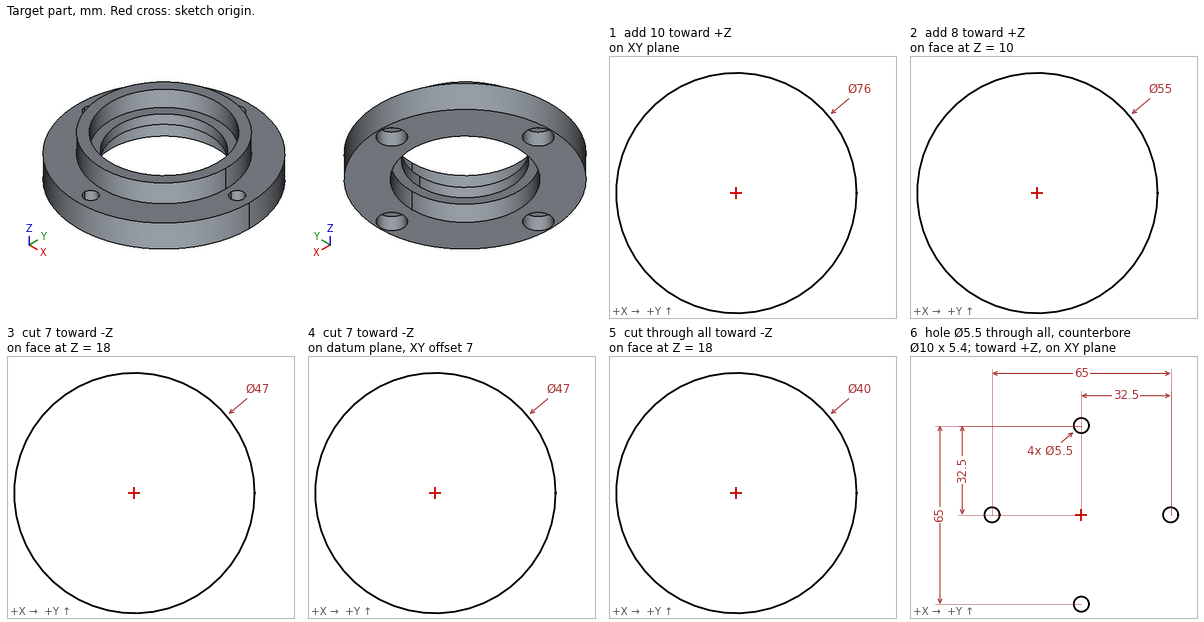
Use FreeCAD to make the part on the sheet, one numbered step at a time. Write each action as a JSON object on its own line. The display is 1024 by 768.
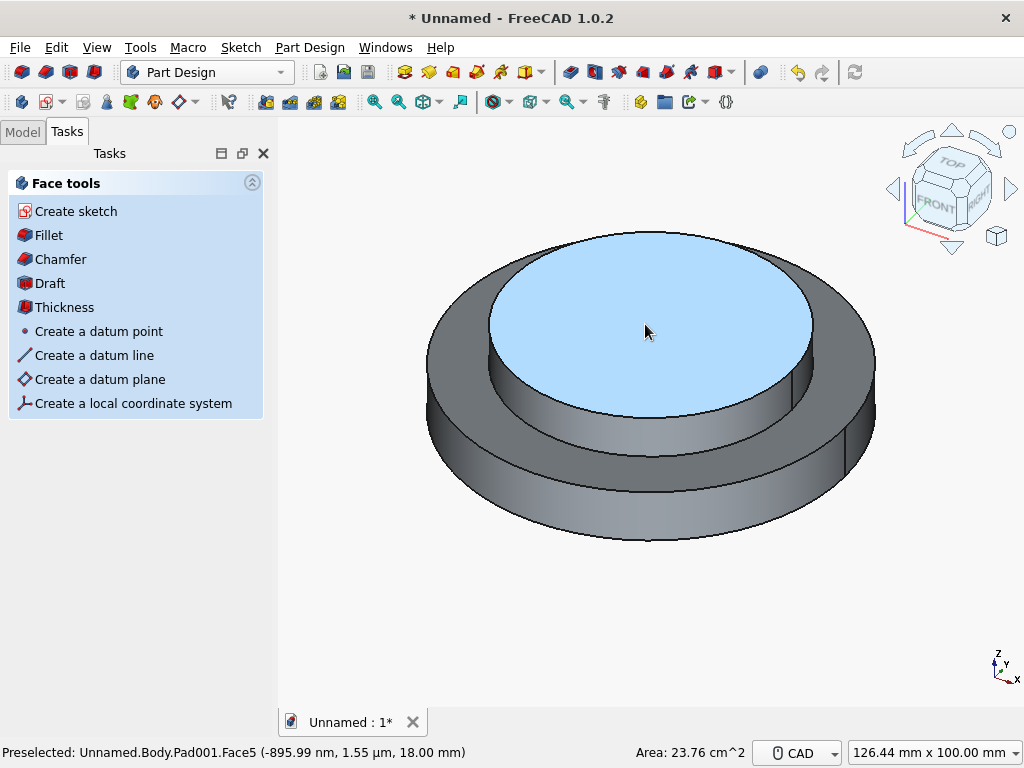
{"action": "left_click", "coordinate": [46, 102]}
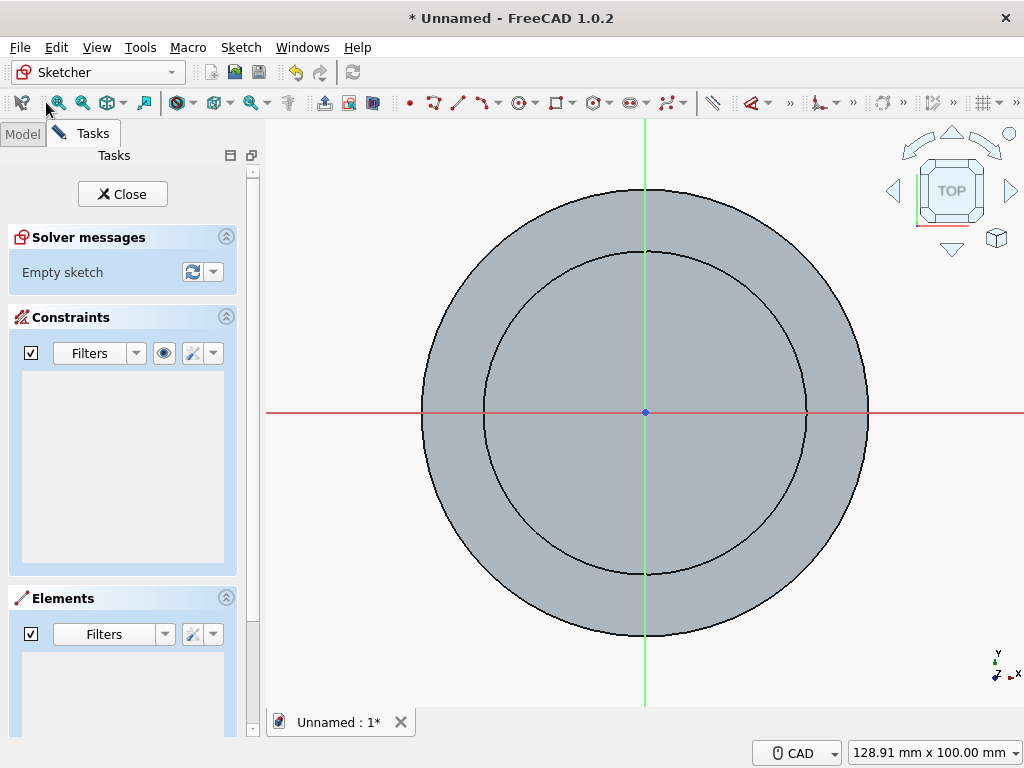
{"action": "scroll", "coordinate": [784, 413], "scroll_direction": "up", "scroll_amount": 2}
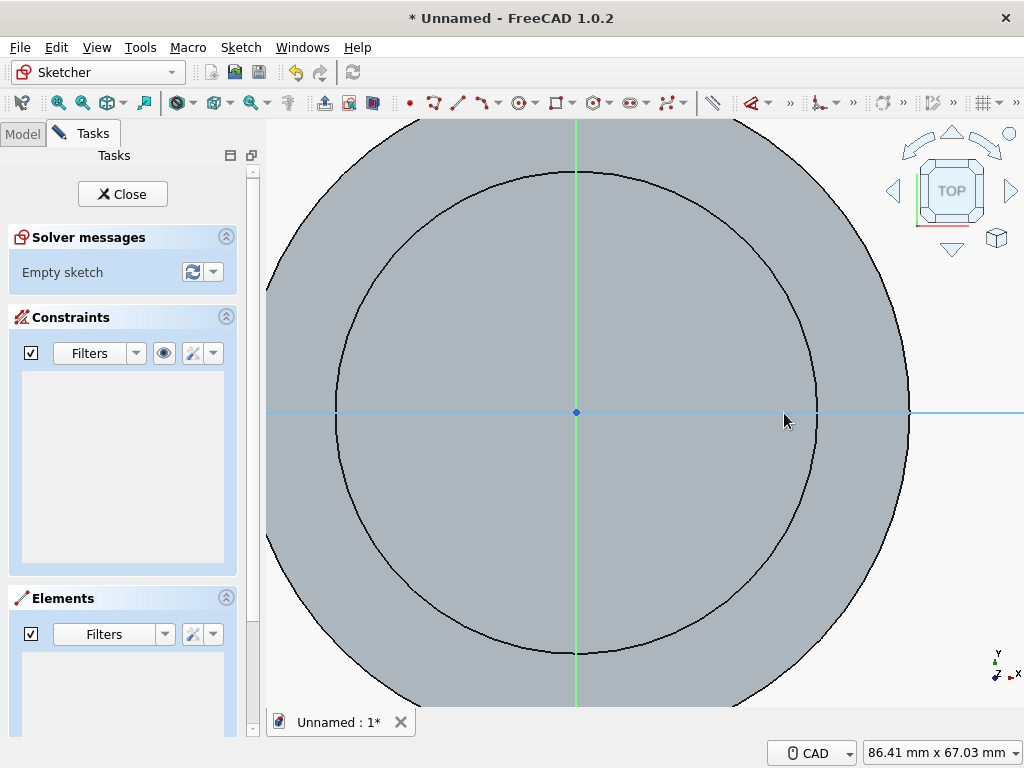
{"action": "key", "text": "g c"}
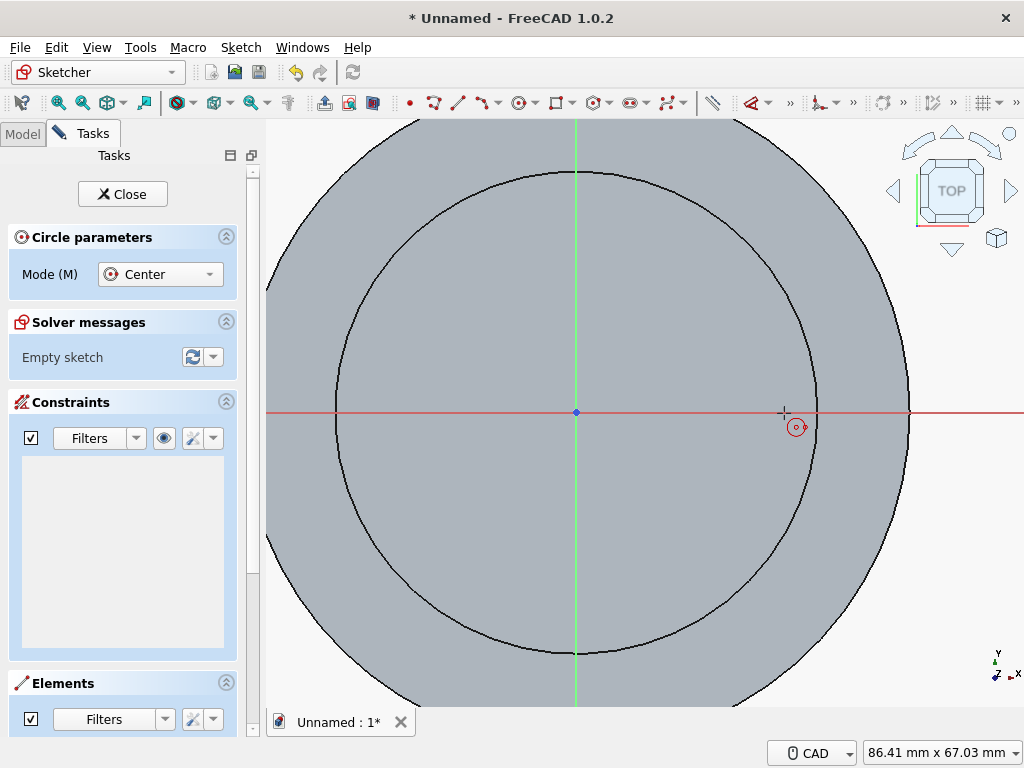
{"action": "left_click", "coordinate": [576, 413]}
{"action": "left_click", "coordinate": [722, 267]}
{"action": "key", "text": "Escape"}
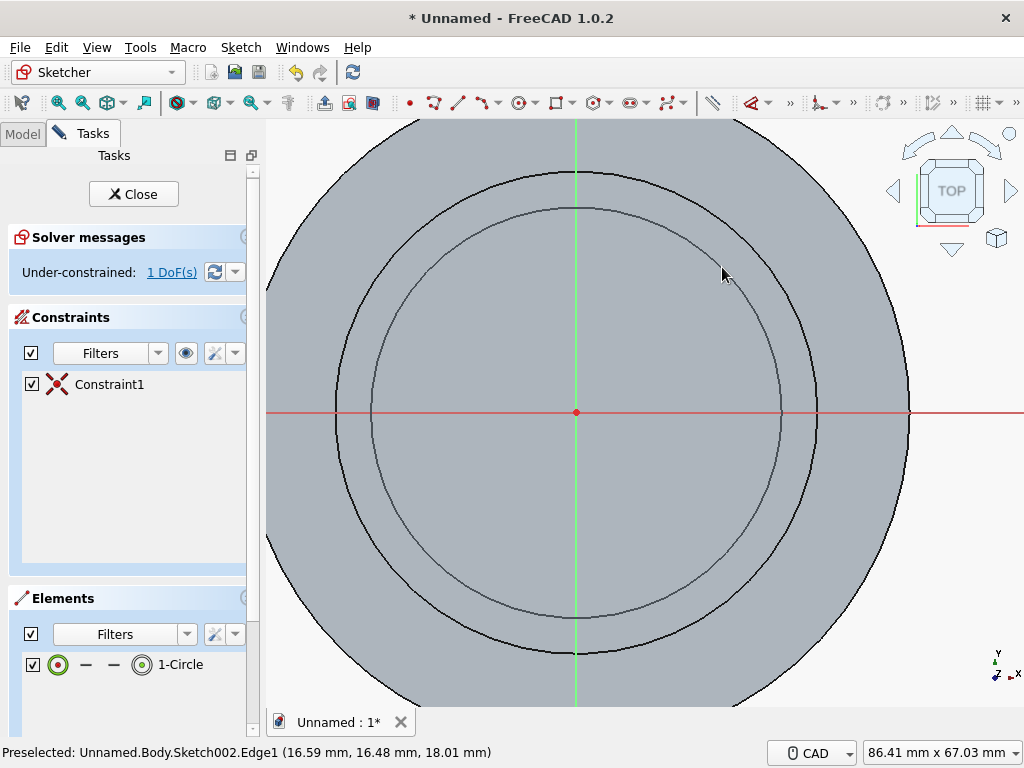
{"action": "left_click", "coordinate": [721, 267]}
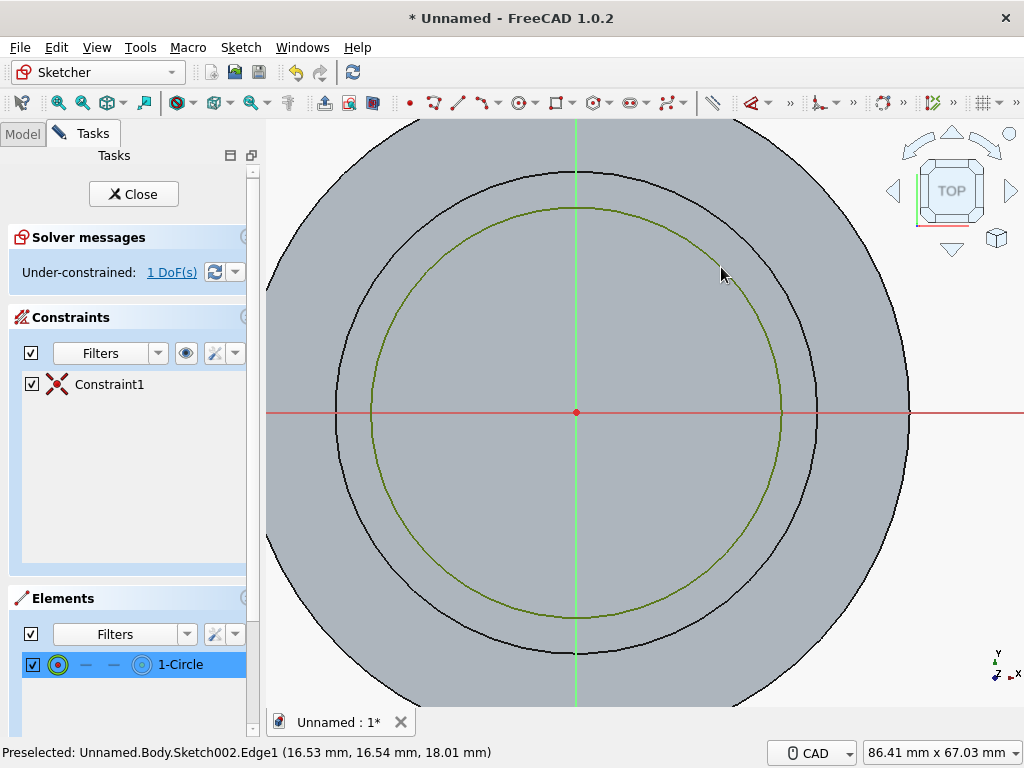
{"action": "key", "text": "k o"}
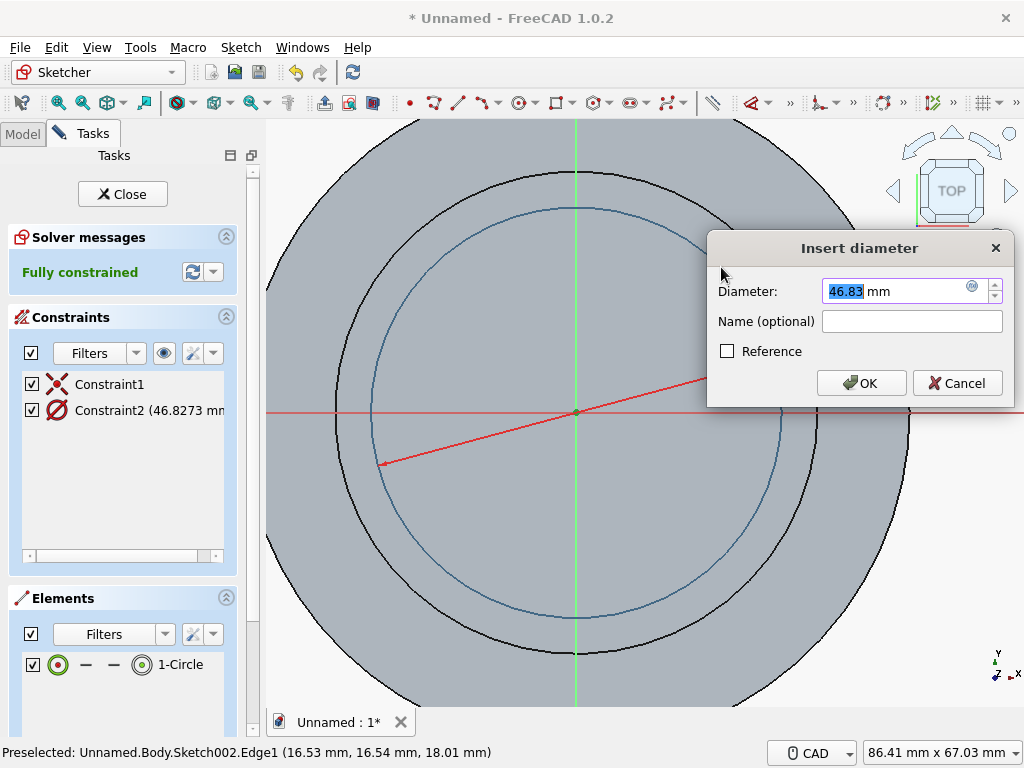
{"action": "type", "text": "47"}
{"action": "key", "text": "Return"}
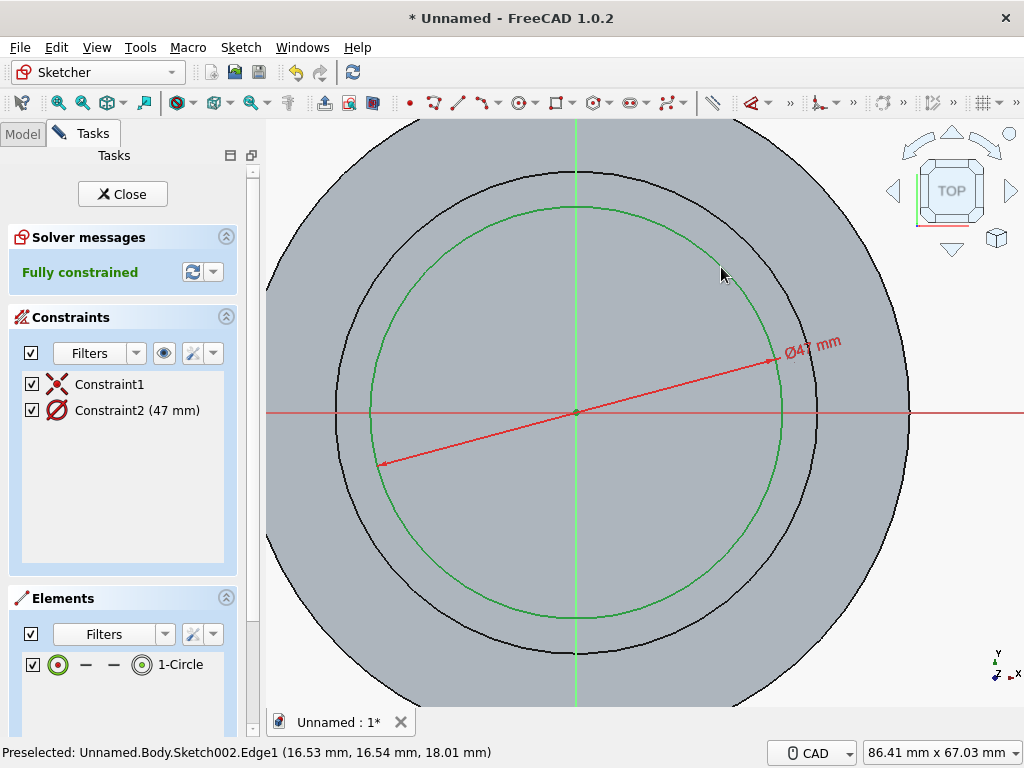
{"action": "left_click", "coordinate": [123, 194]}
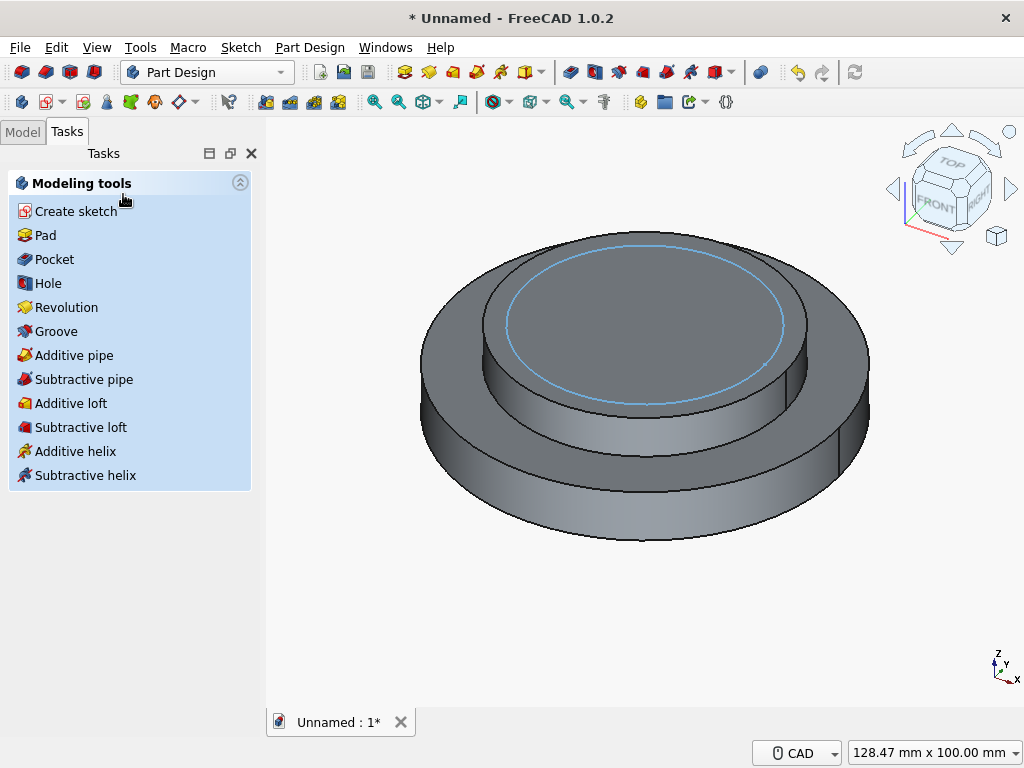
{"action": "left_click", "coordinate": [572, 72]}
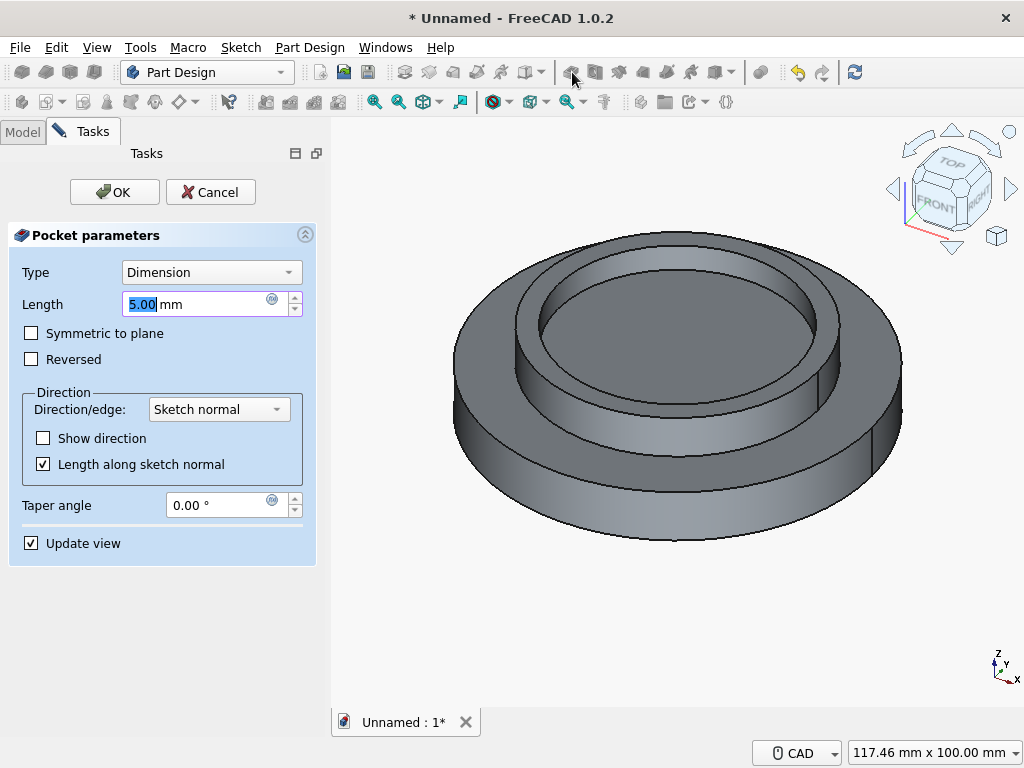
{"action": "type", "text": "7"}
{"action": "key", "text": "Tab"}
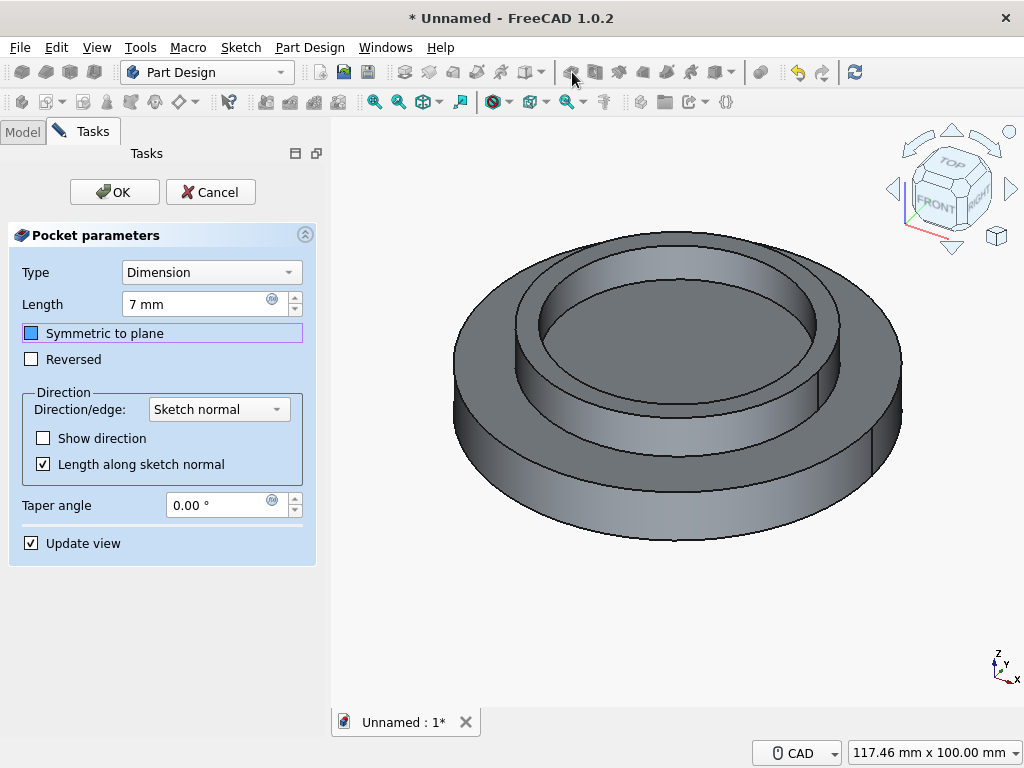
{"action": "left_click", "coordinate": [115, 192]}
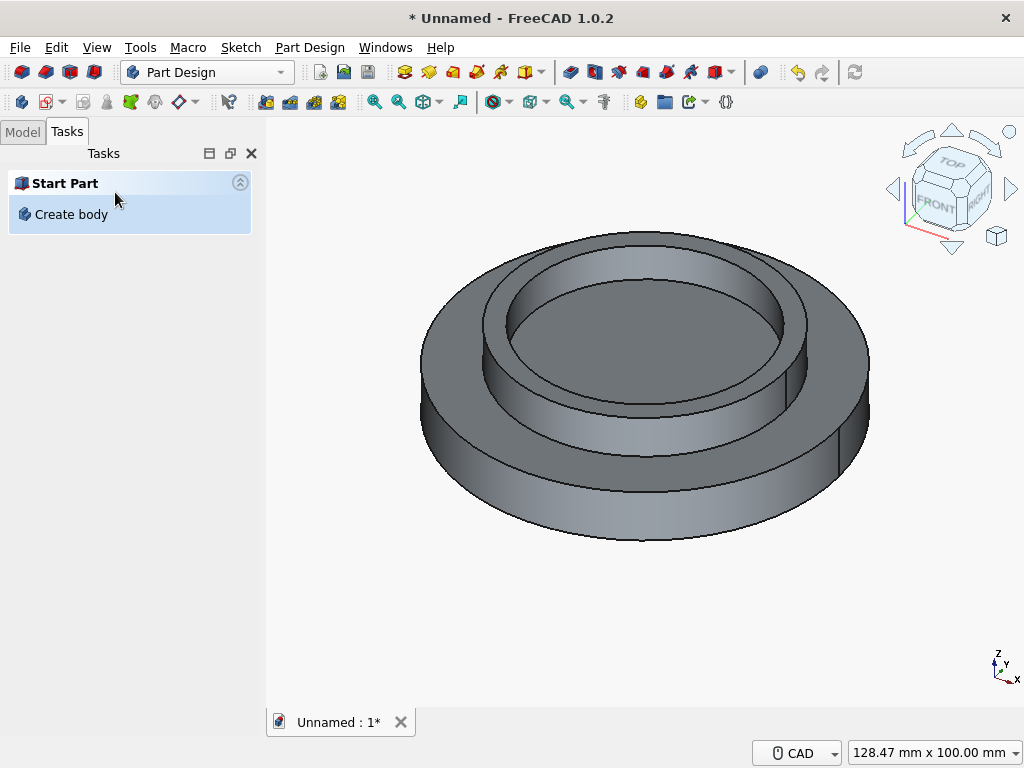
{"action": "left_click", "coordinate": [23, 131]}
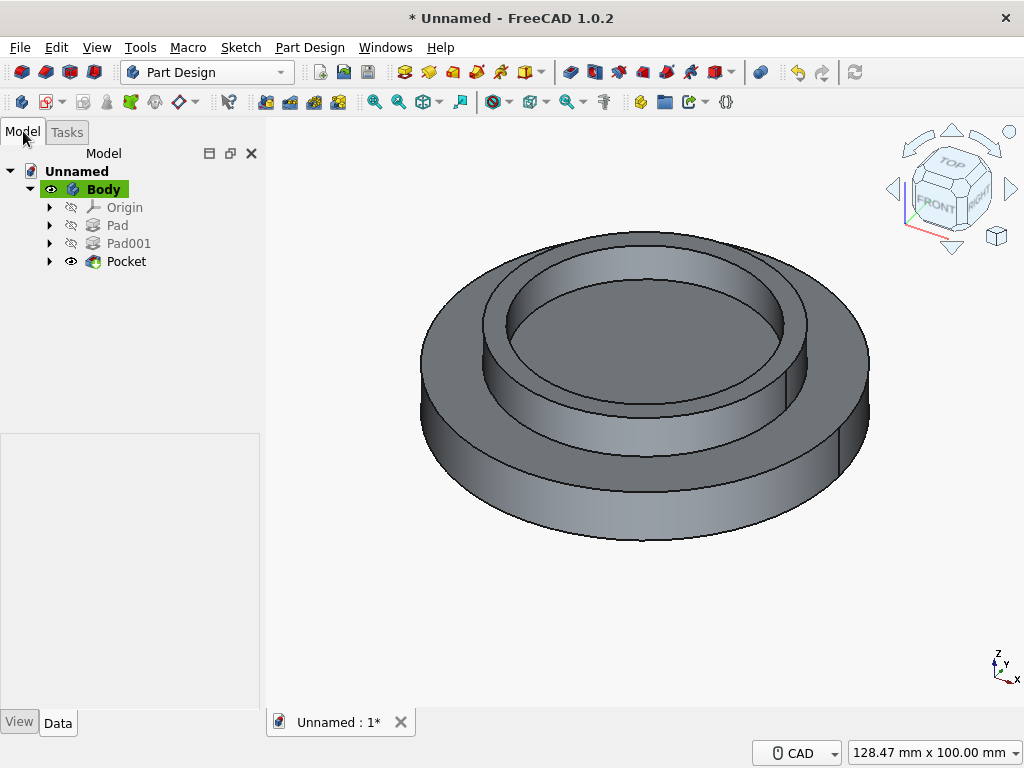
{"action": "left_click", "coordinate": [50, 207]}